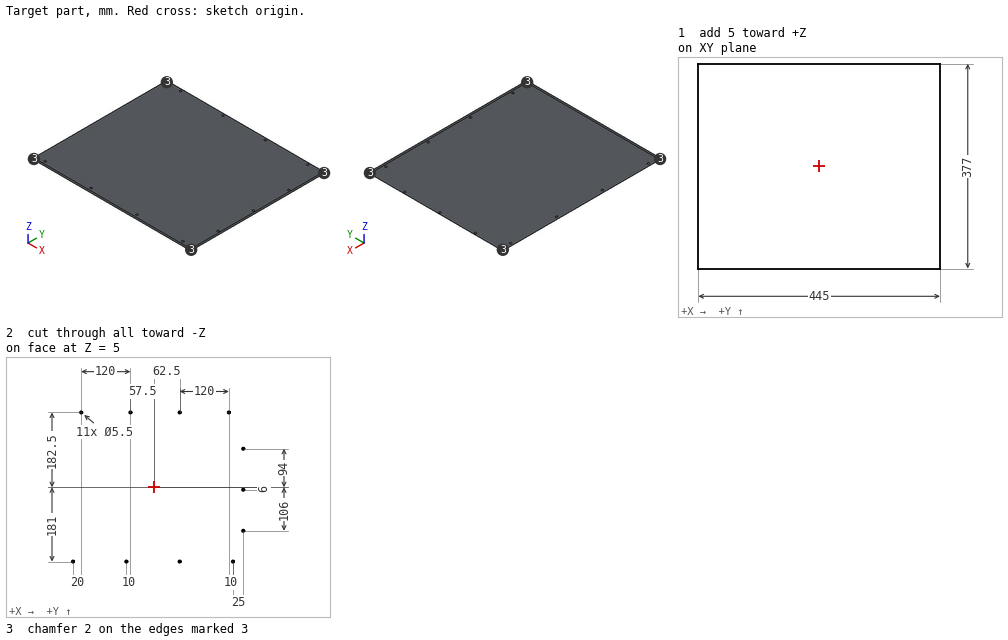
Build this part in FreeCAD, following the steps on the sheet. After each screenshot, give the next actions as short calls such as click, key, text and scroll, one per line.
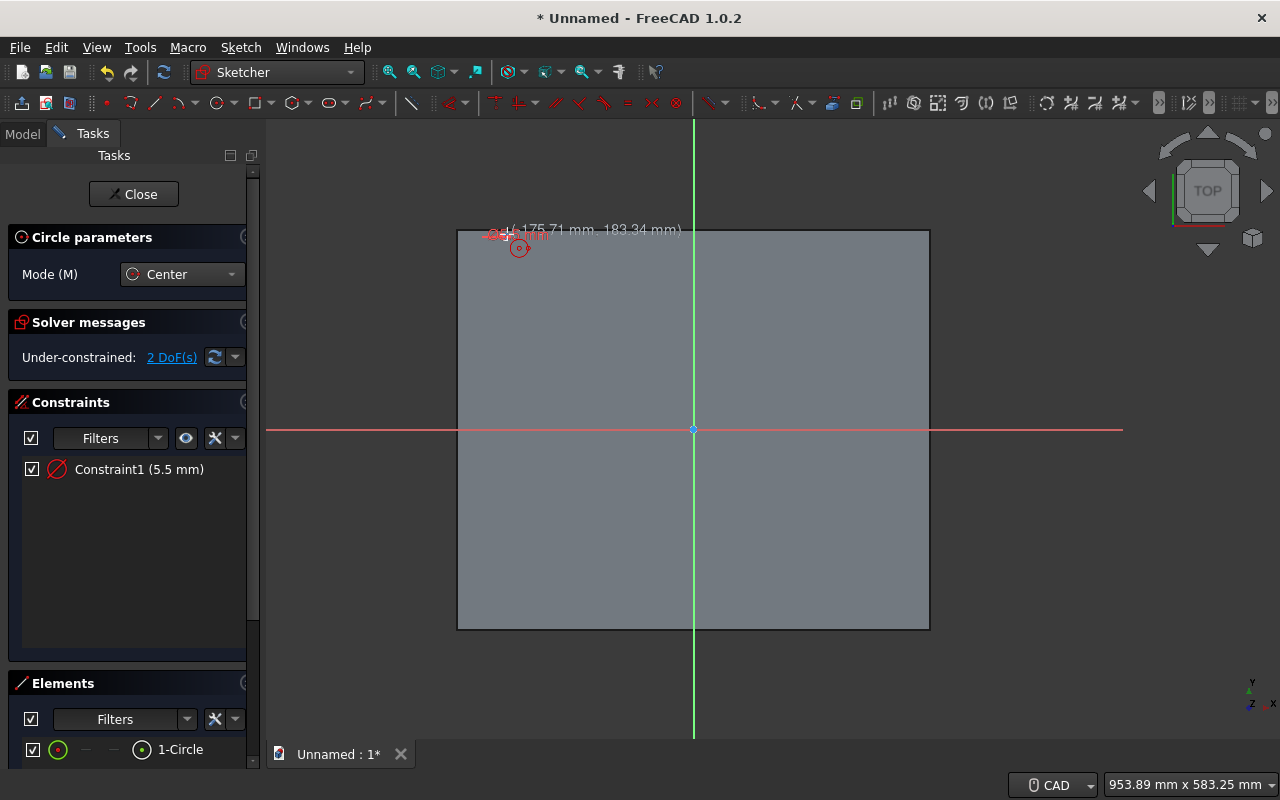
scroll(633, 236, up, 11)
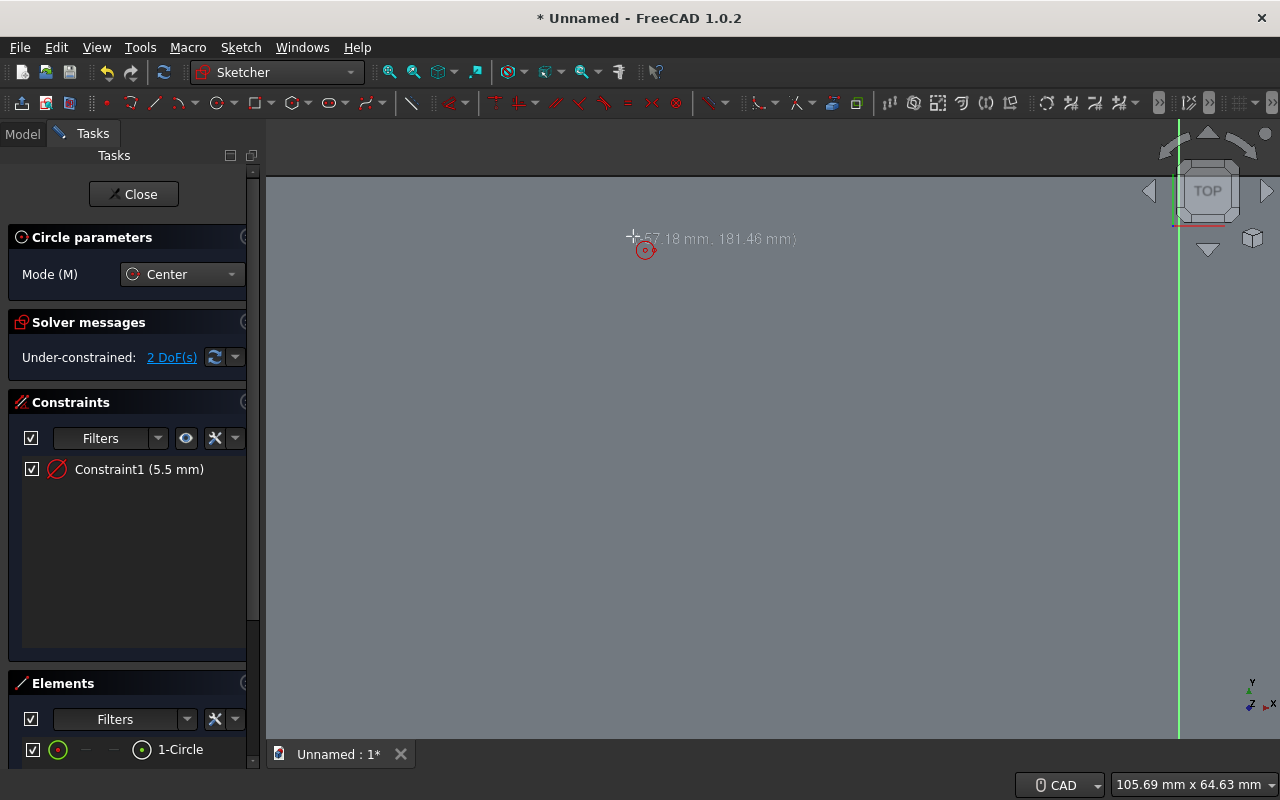
scroll(633, 236, down, 11)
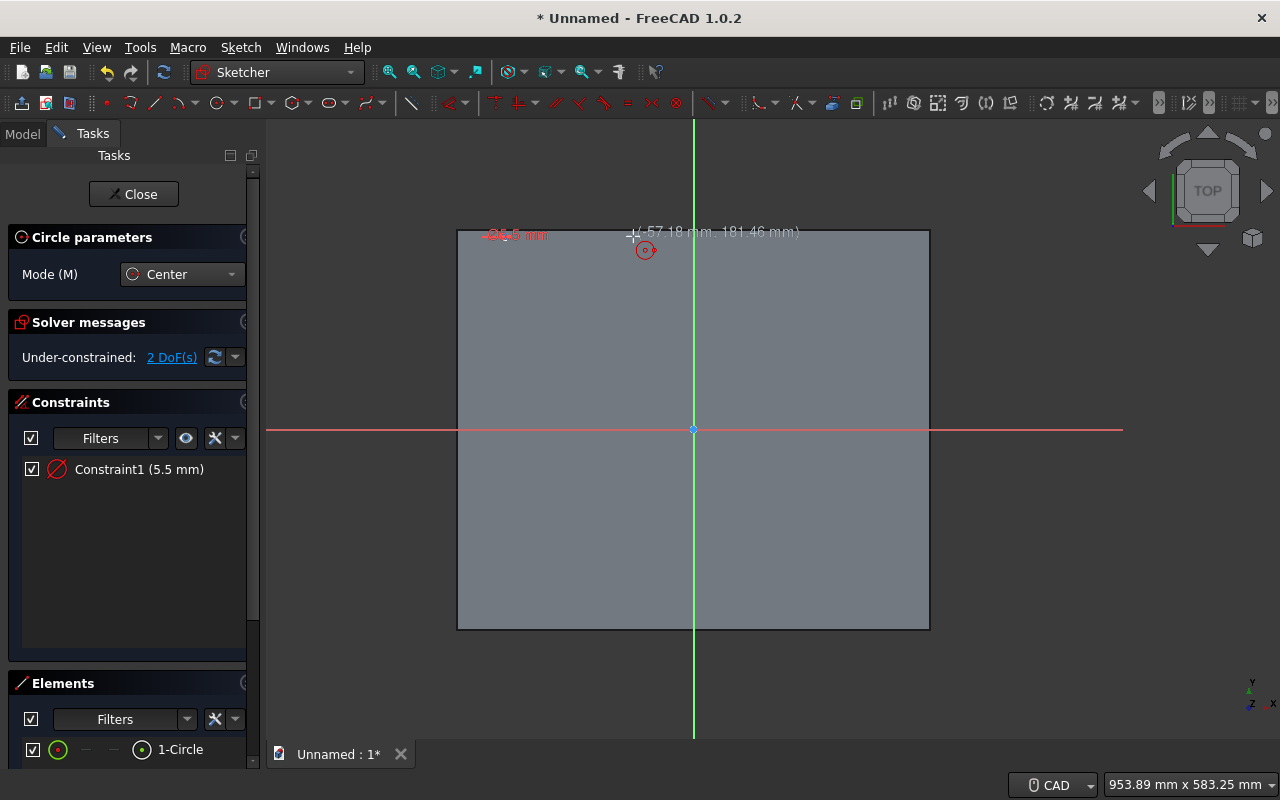
click(633, 236)
move(635, 234)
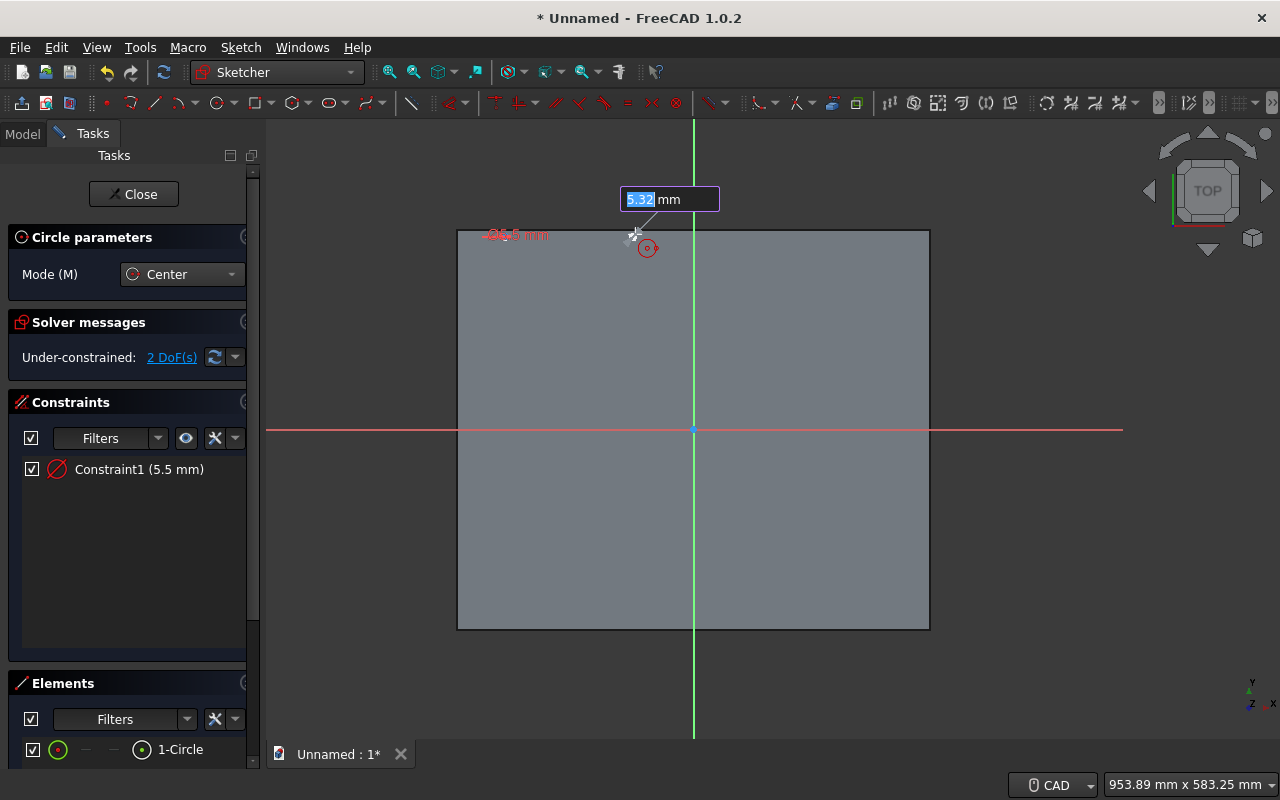
text(5.5)
key(Return)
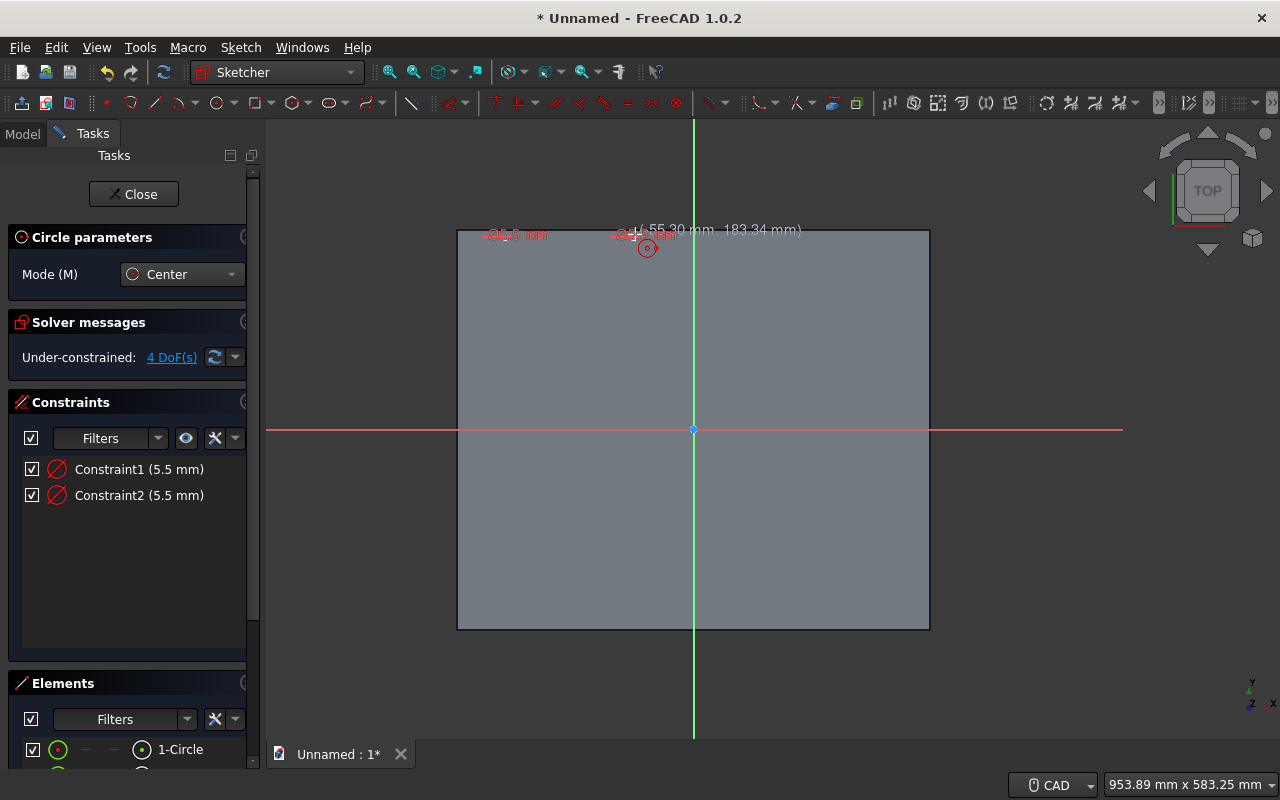
scroll(760, 236, up, 11)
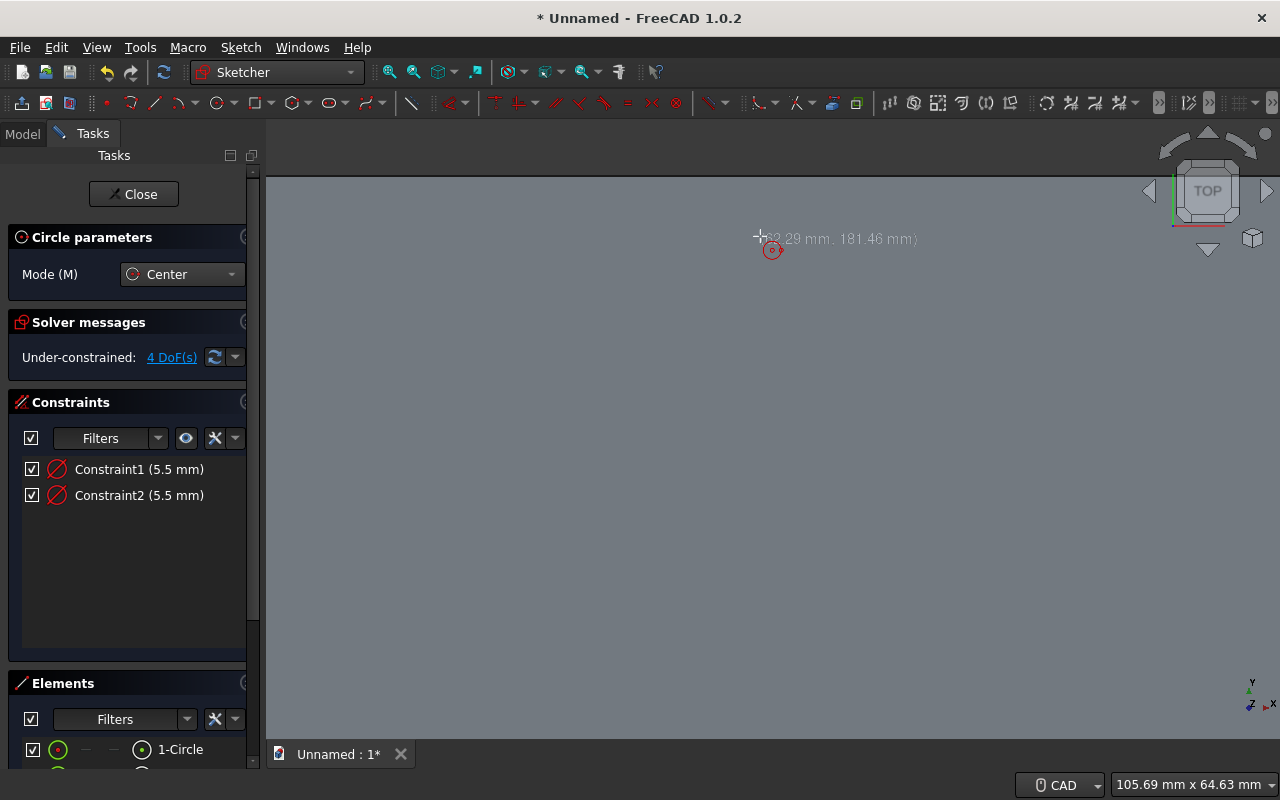
scroll(761, 236, down, 11)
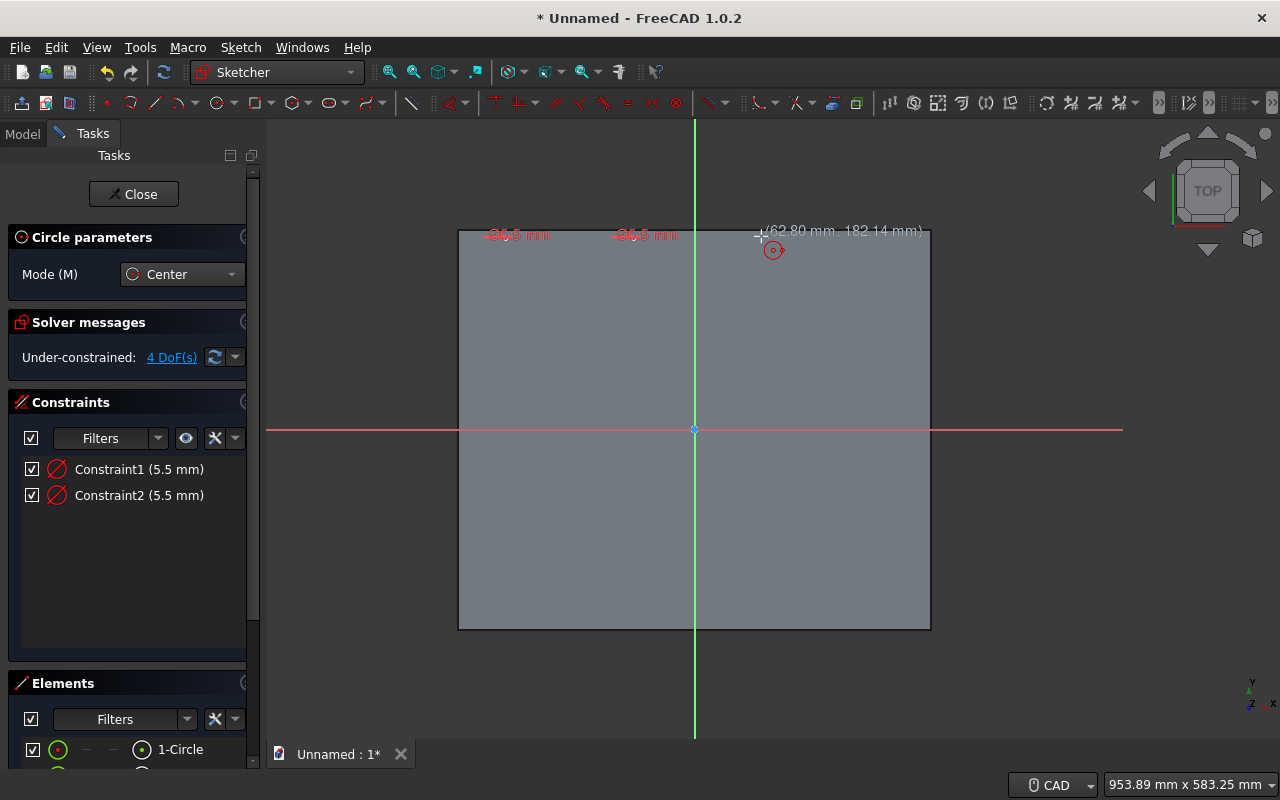
click(761, 236)
move(763, 234)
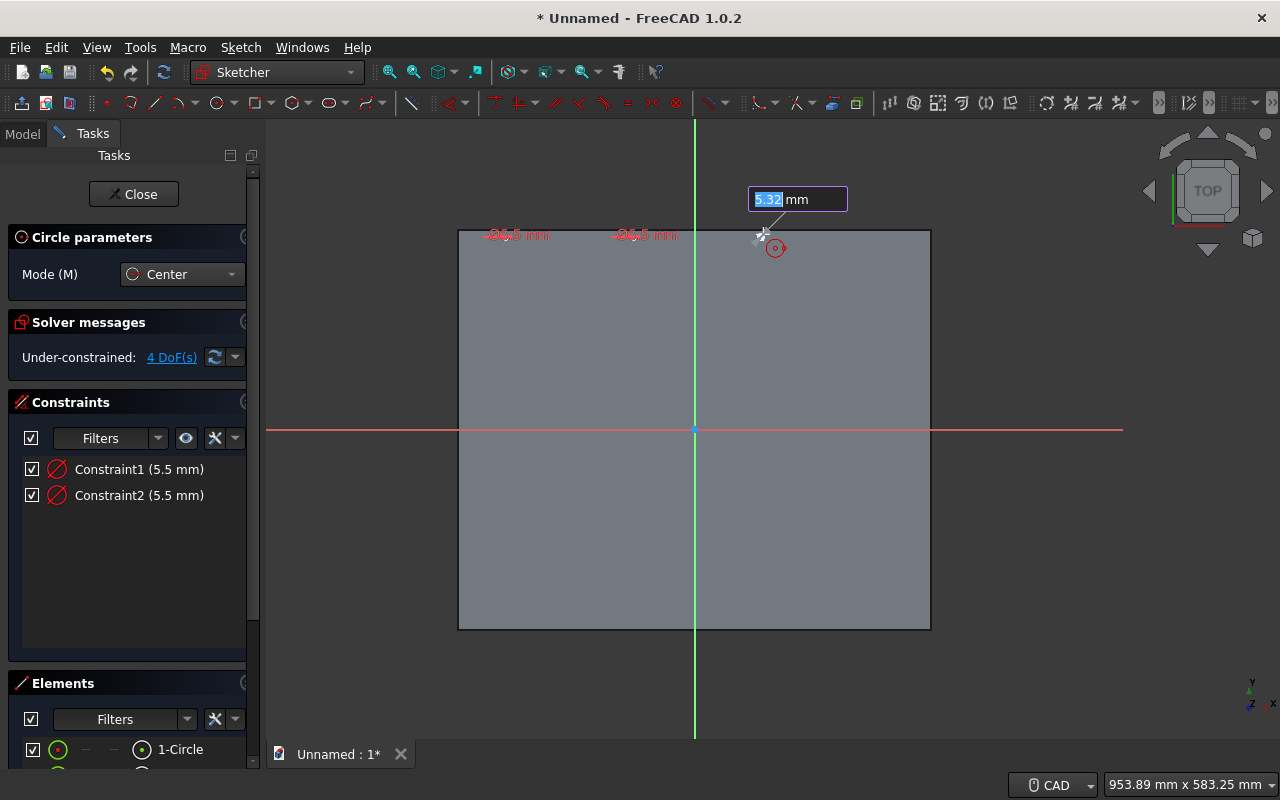
text(5.5)
key(Return)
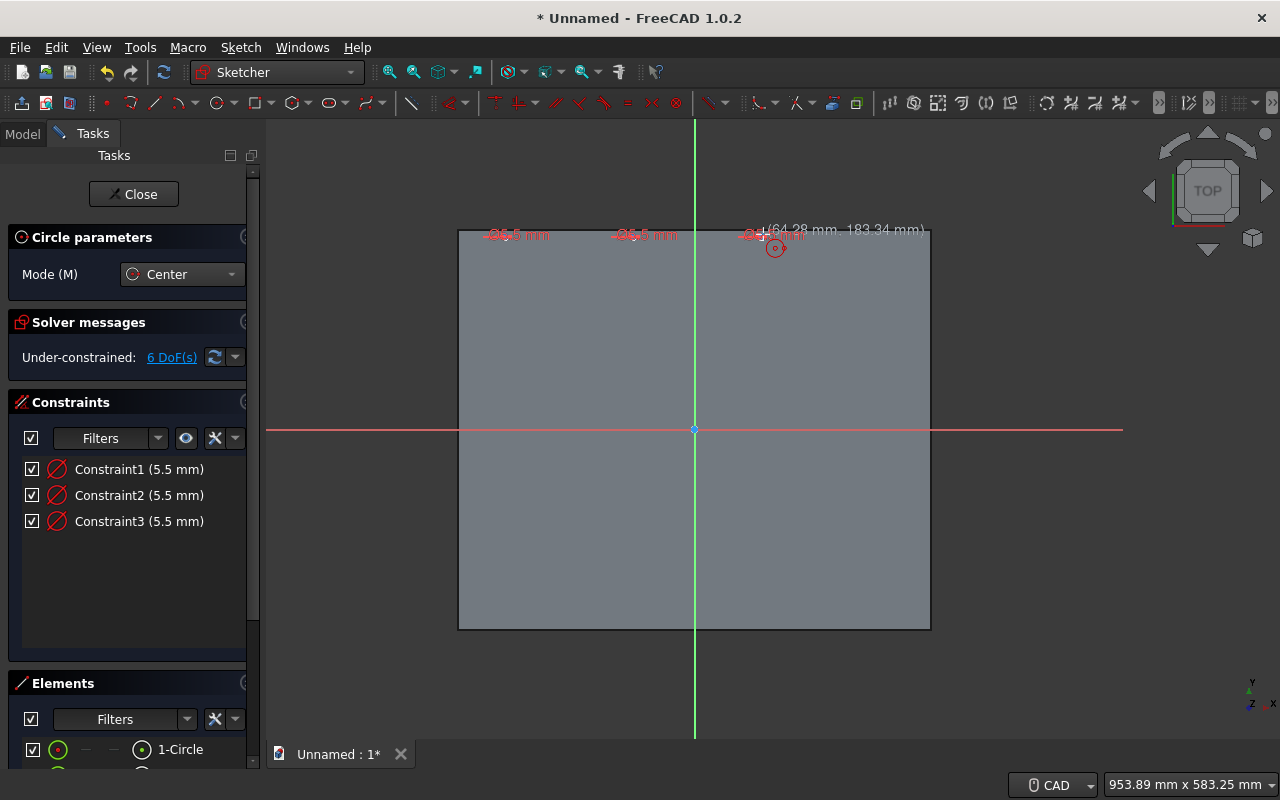
scroll(889, 236, up, 11)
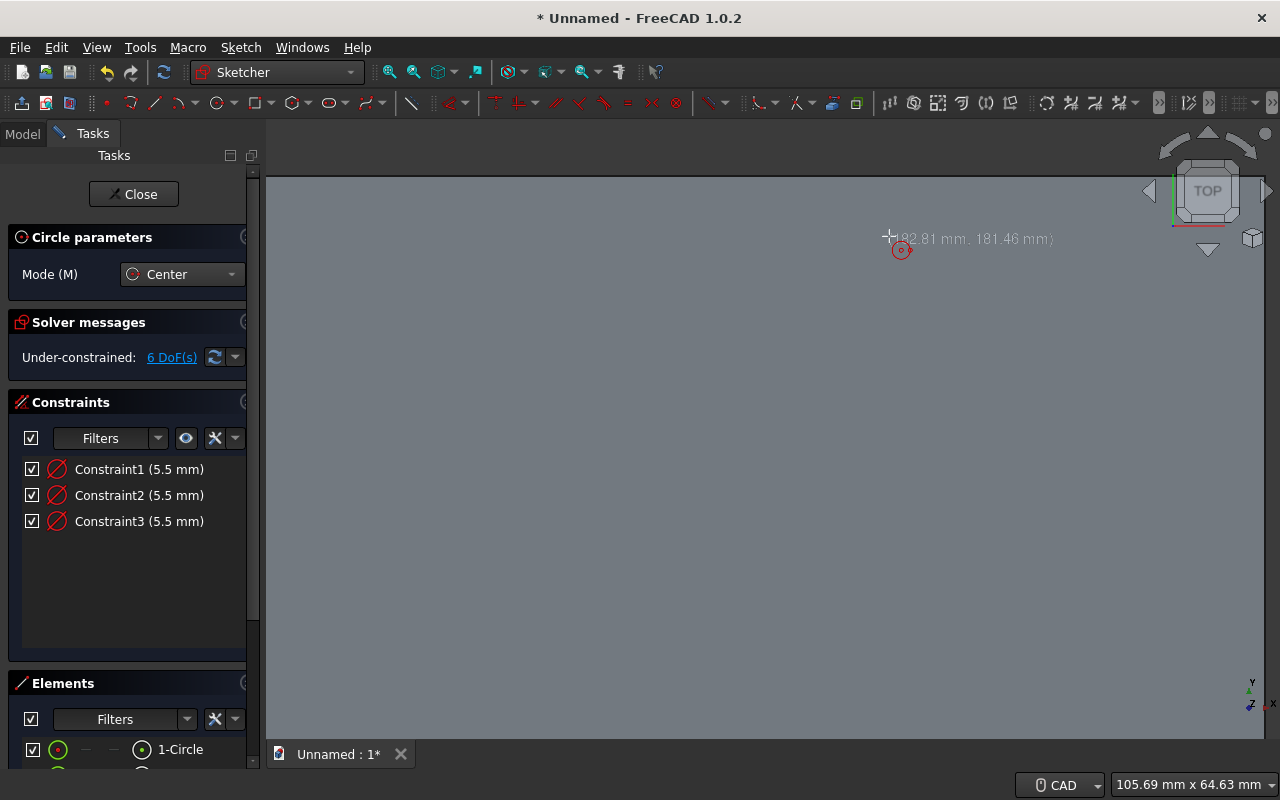
scroll(889, 236, down, 11)